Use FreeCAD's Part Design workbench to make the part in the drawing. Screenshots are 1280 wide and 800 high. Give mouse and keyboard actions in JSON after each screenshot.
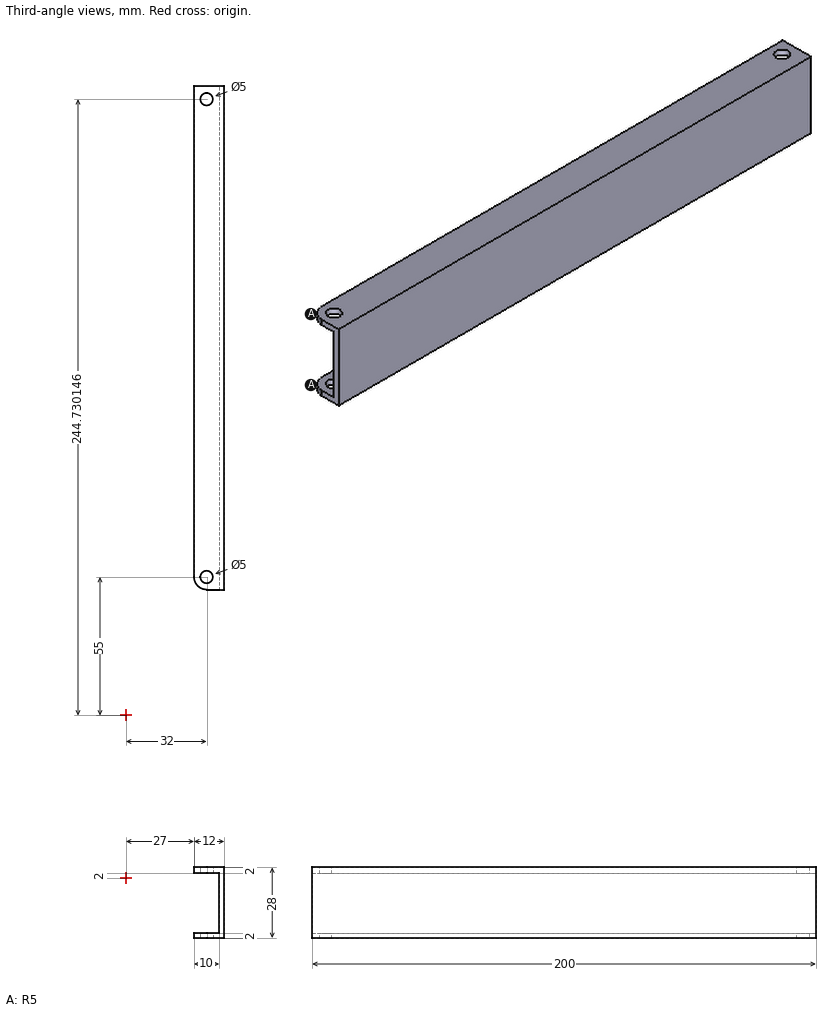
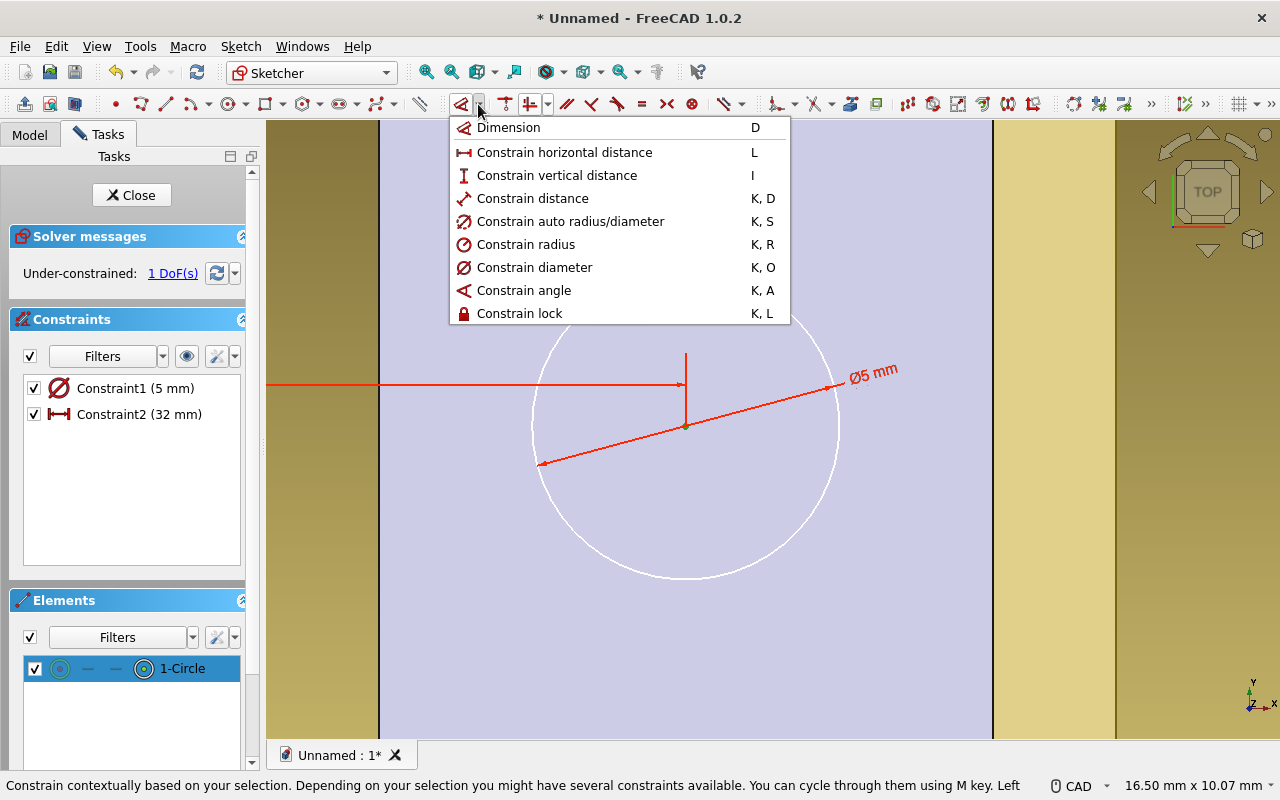
{"action": "left_click", "coordinate": [620, 176]}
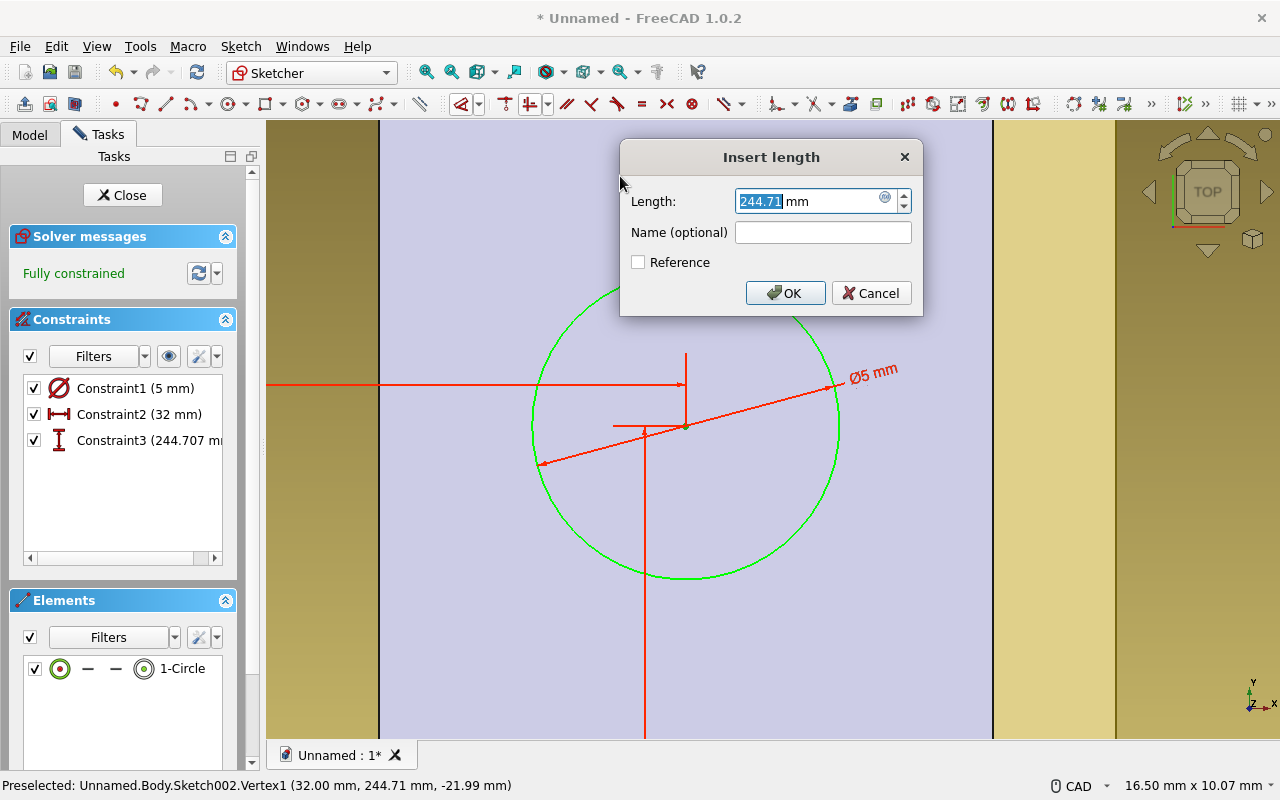
{"action": "type", "text": "244.730146"}
{"action": "key", "text": "Return"}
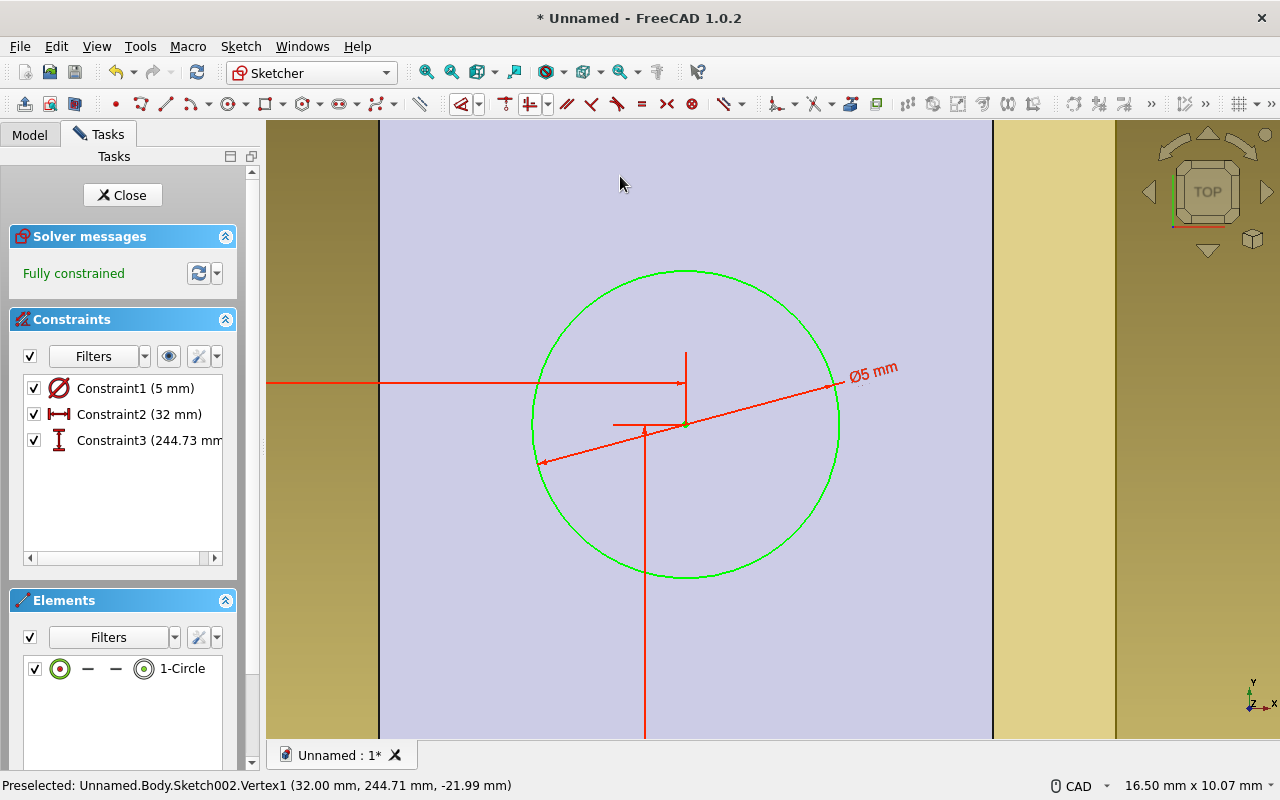
{"action": "left_click", "coordinate": [123, 195]}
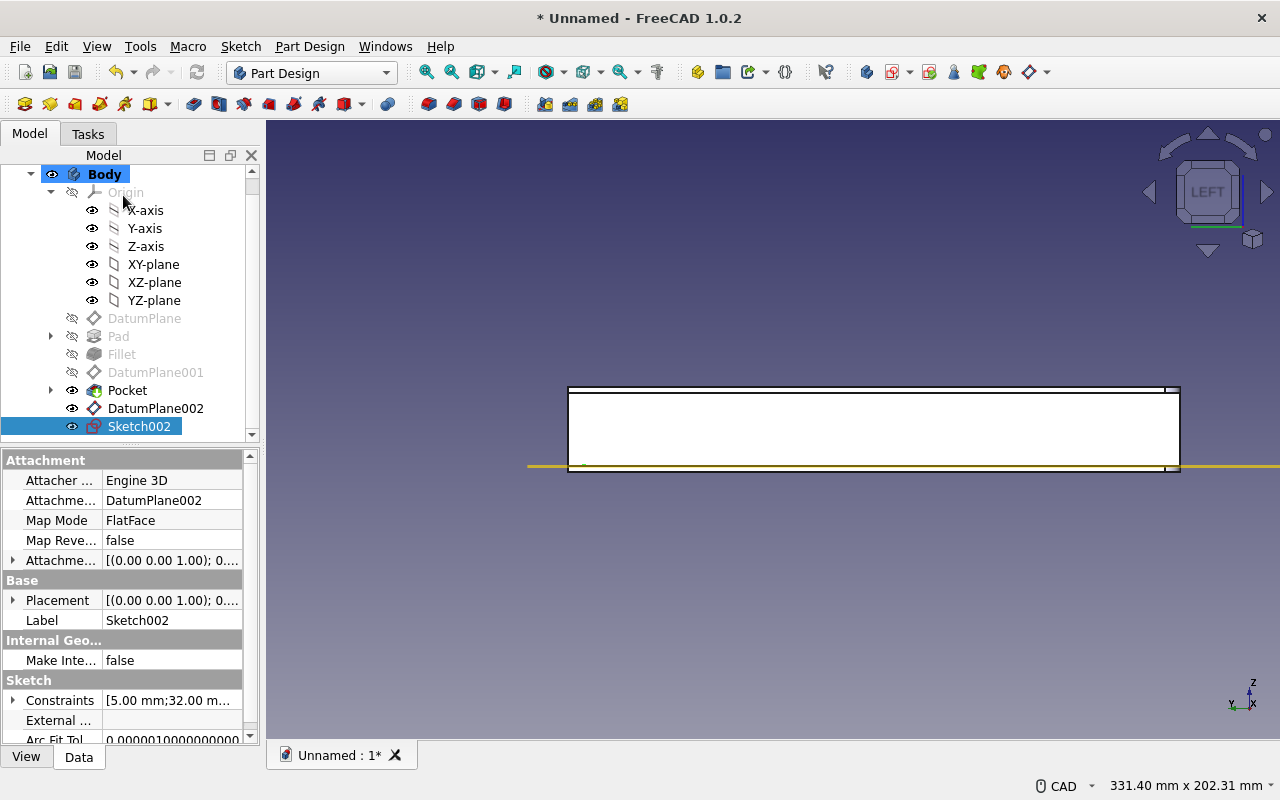
{"action": "left_click", "coordinate": [194, 104]}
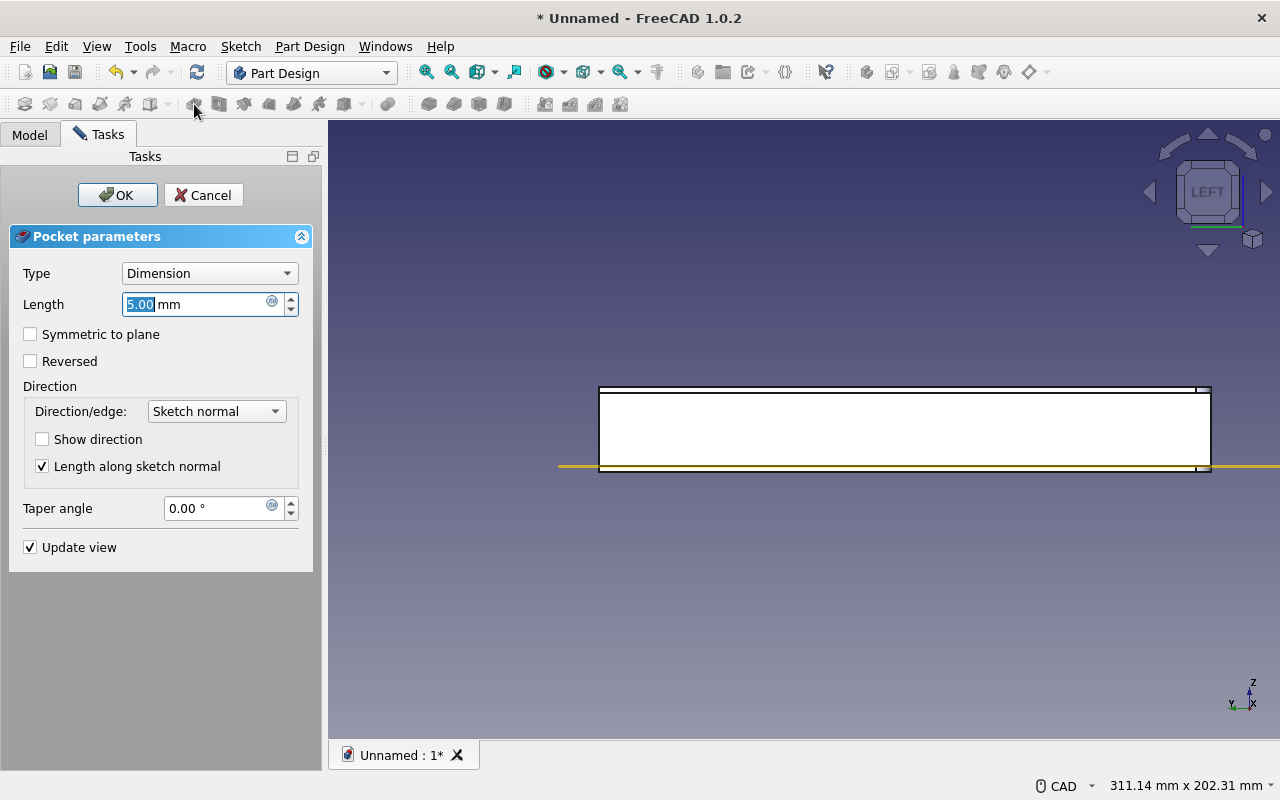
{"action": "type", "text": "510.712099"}
{"action": "key", "text": "Tab"}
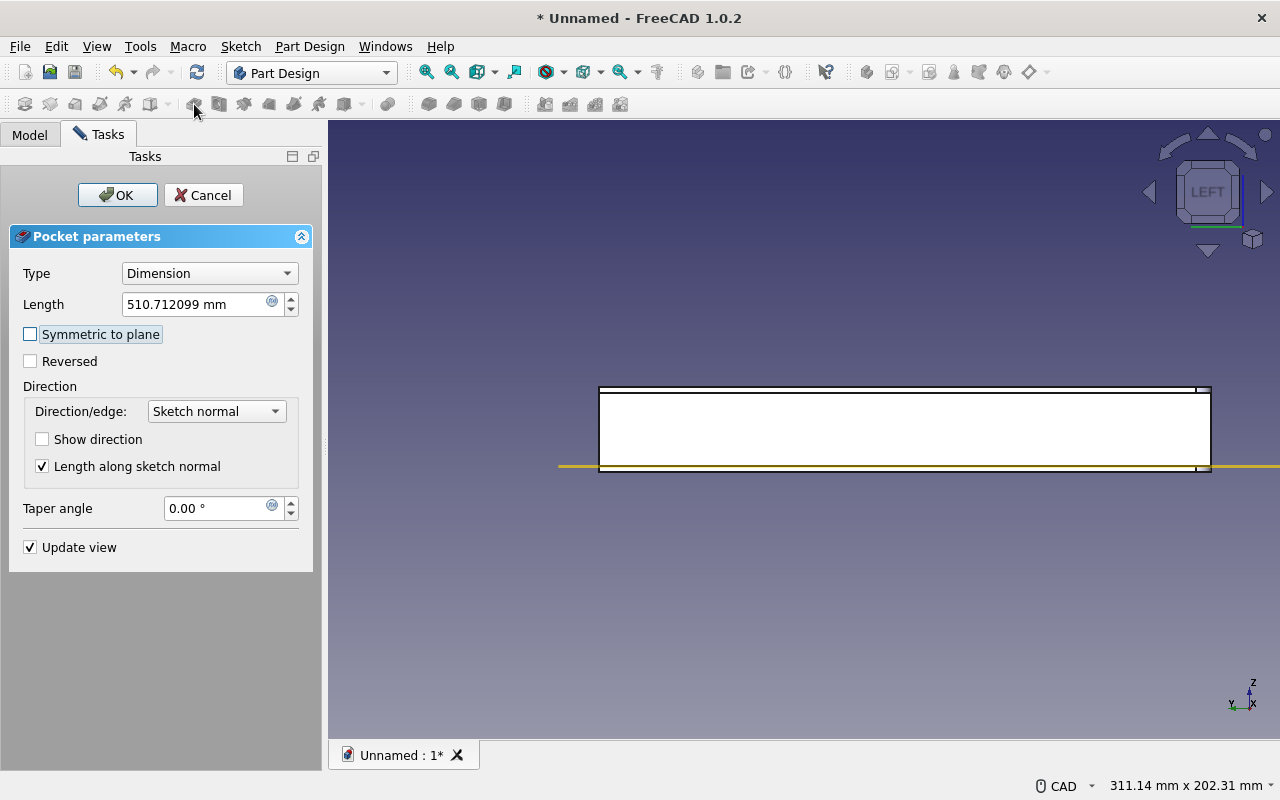
{"action": "left_click", "coordinate": [31, 334]}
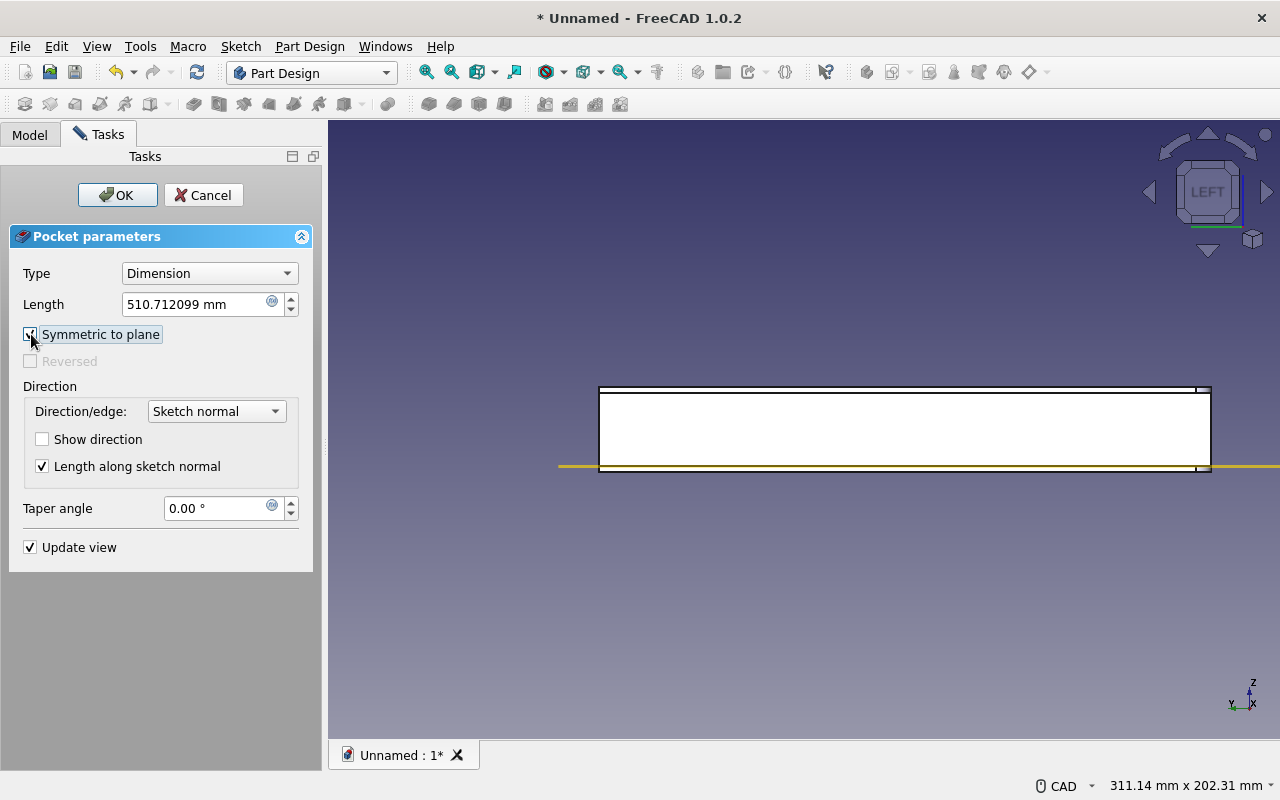
{"action": "left_click", "coordinate": [118, 195]}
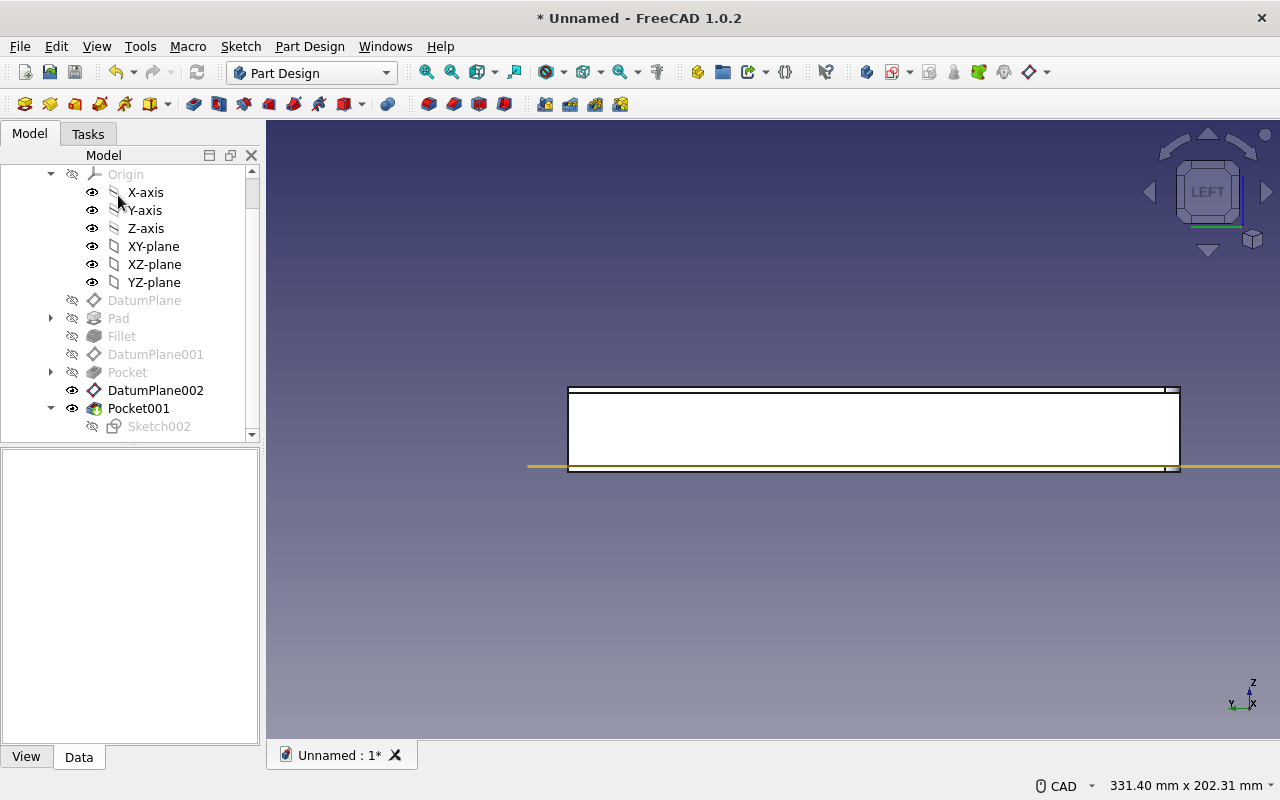
{"action": "left_click", "coordinate": [117, 390]}
{"action": "key", "text": "space"}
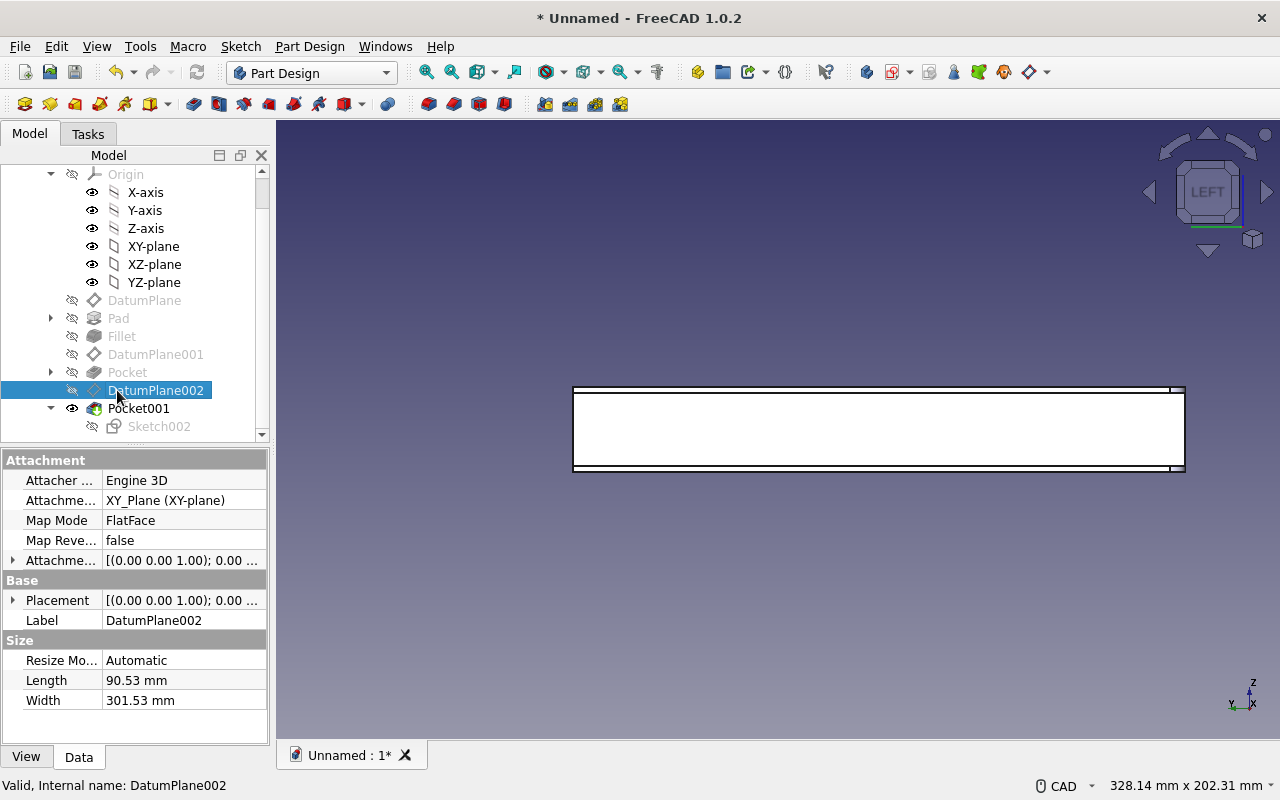
{"action": "key", "text": "0"}